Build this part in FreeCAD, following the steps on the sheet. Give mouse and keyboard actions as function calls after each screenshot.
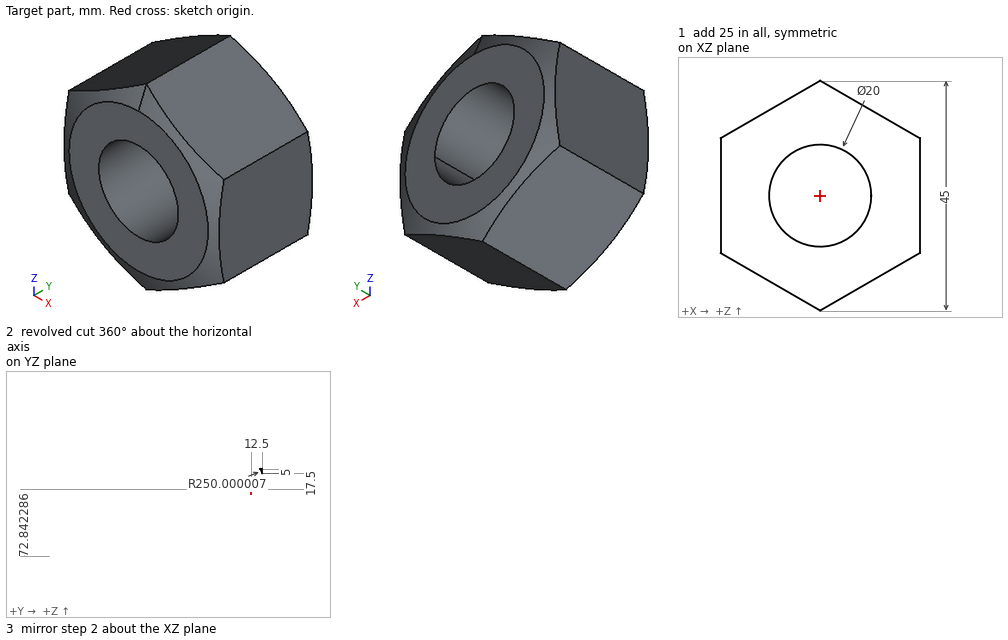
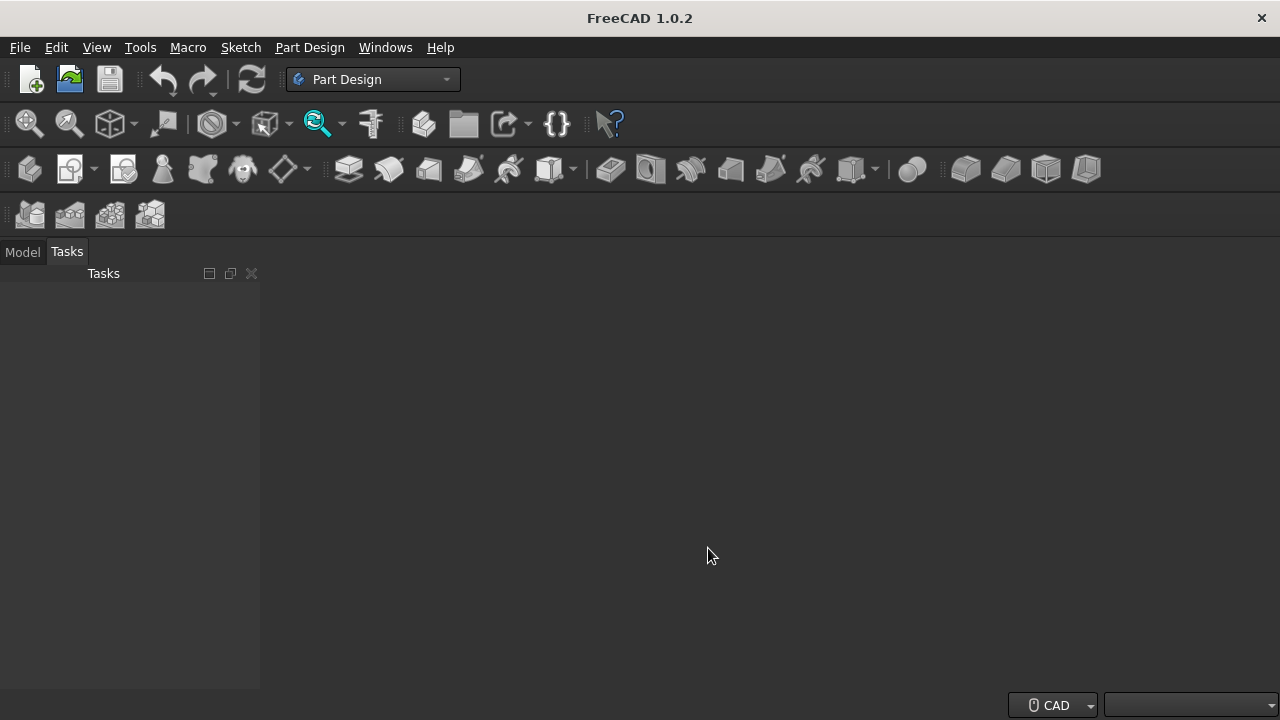
click(30, 80)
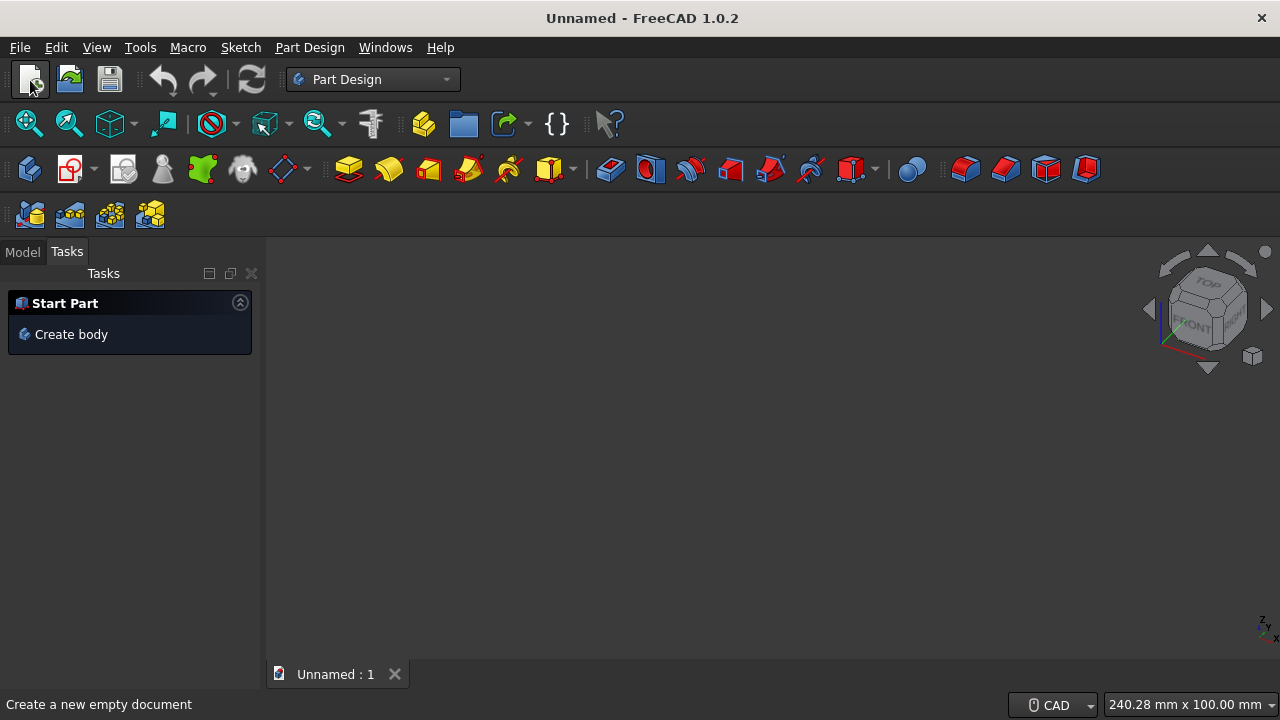
click(70, 170)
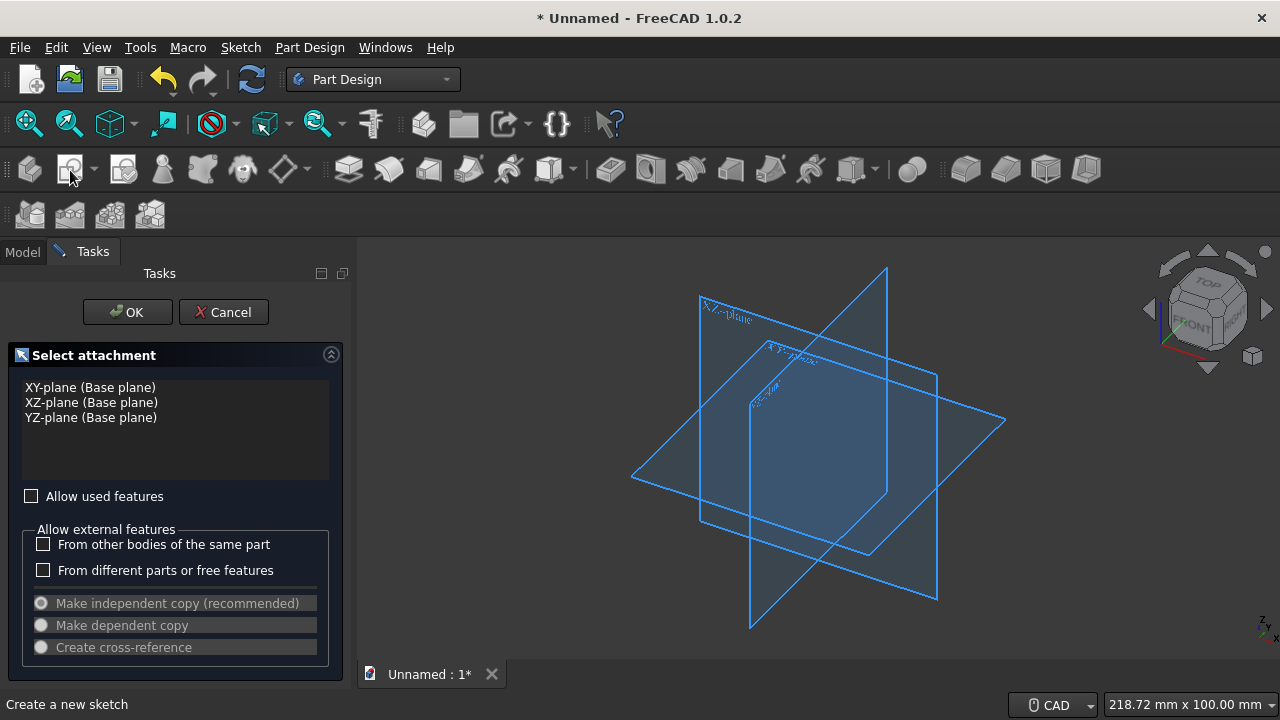
click(82, 402)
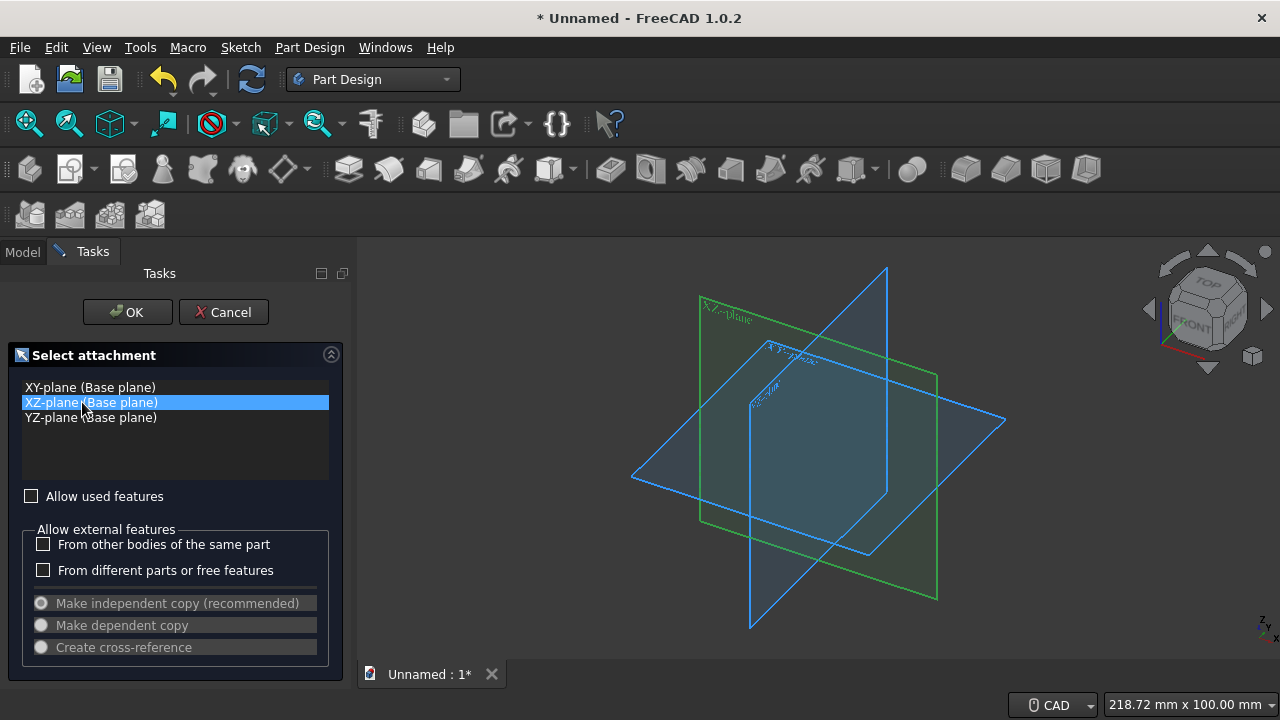
click(128, 312)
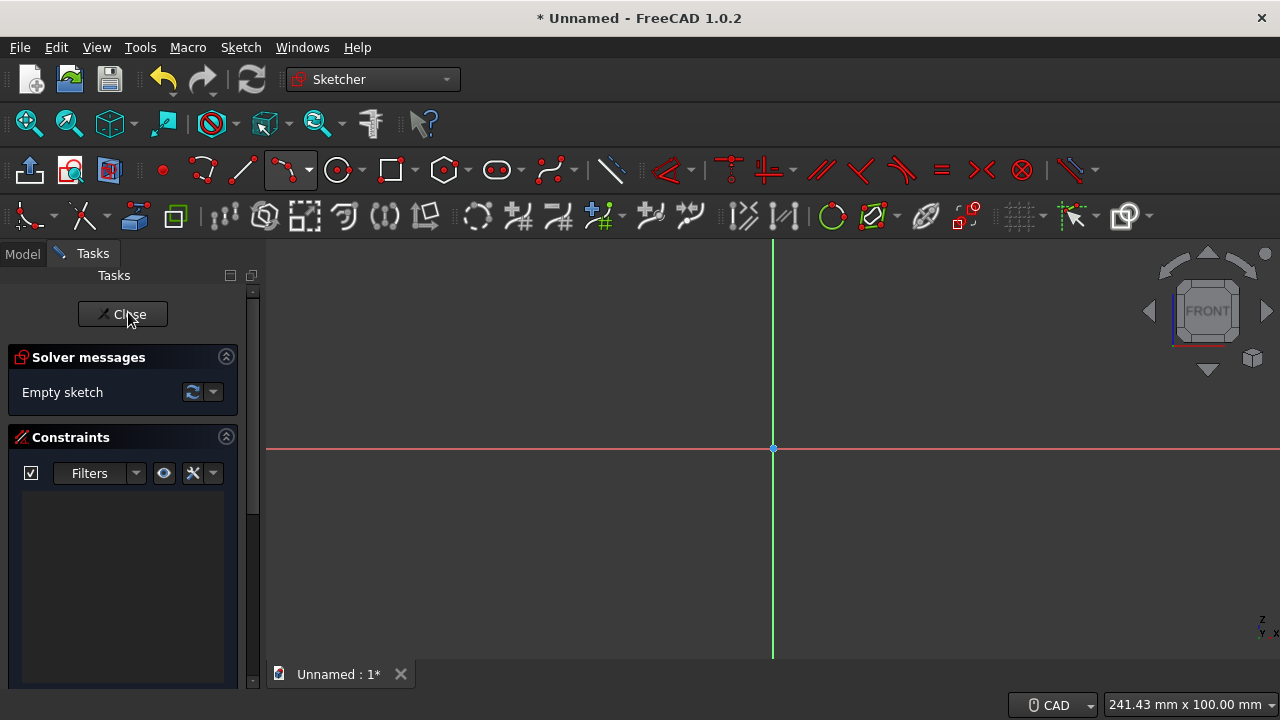
scroll(912, 449, up, 2)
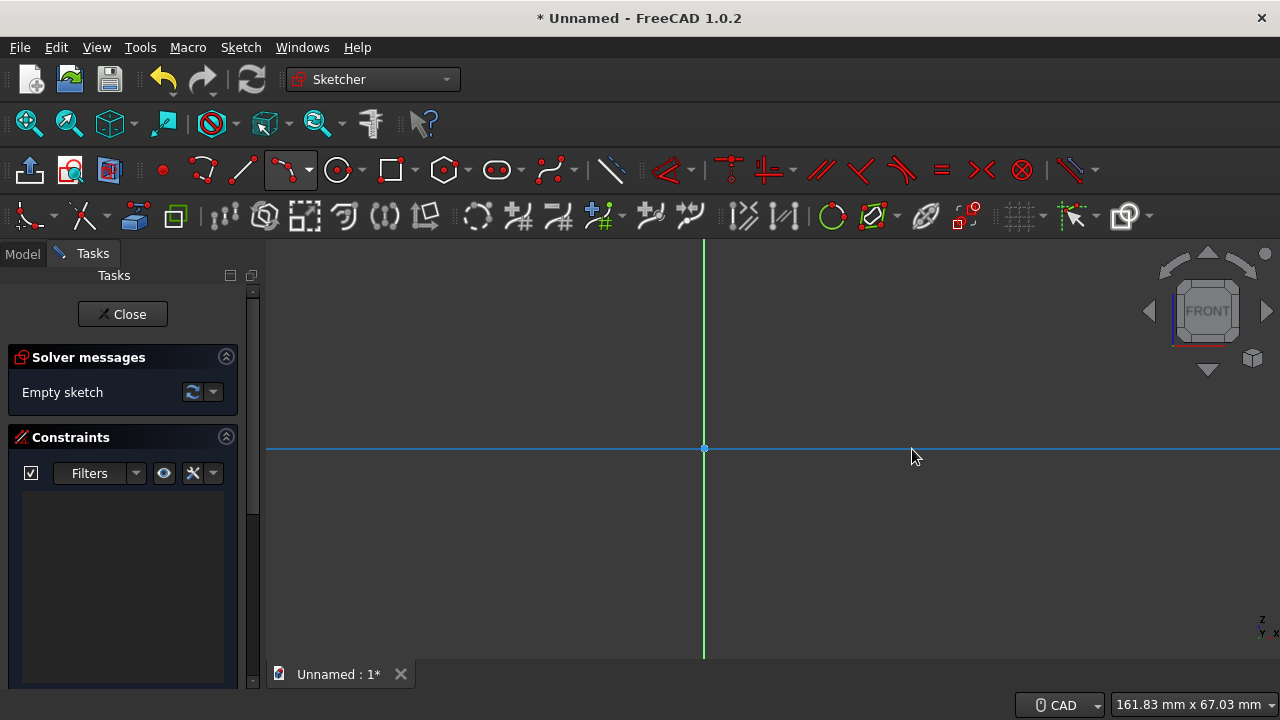
click(444, 170)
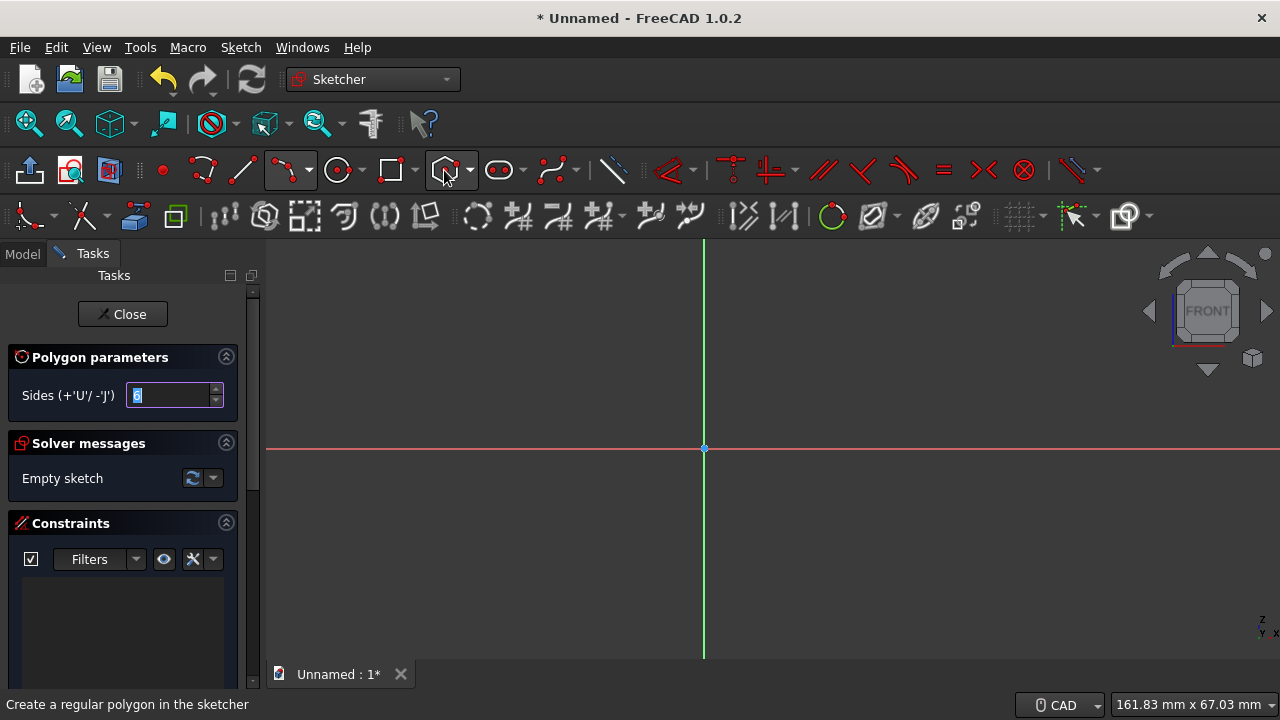
click(704, 449)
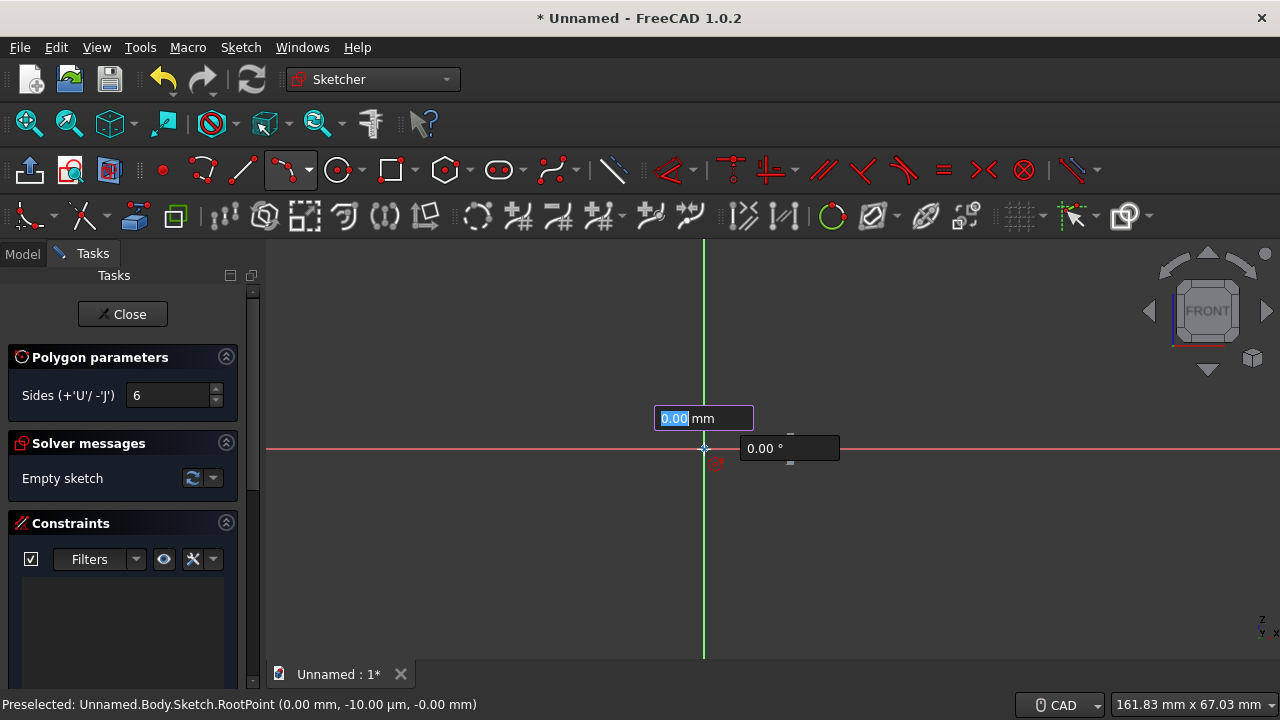
click(704, 590)
right_click(704, 590)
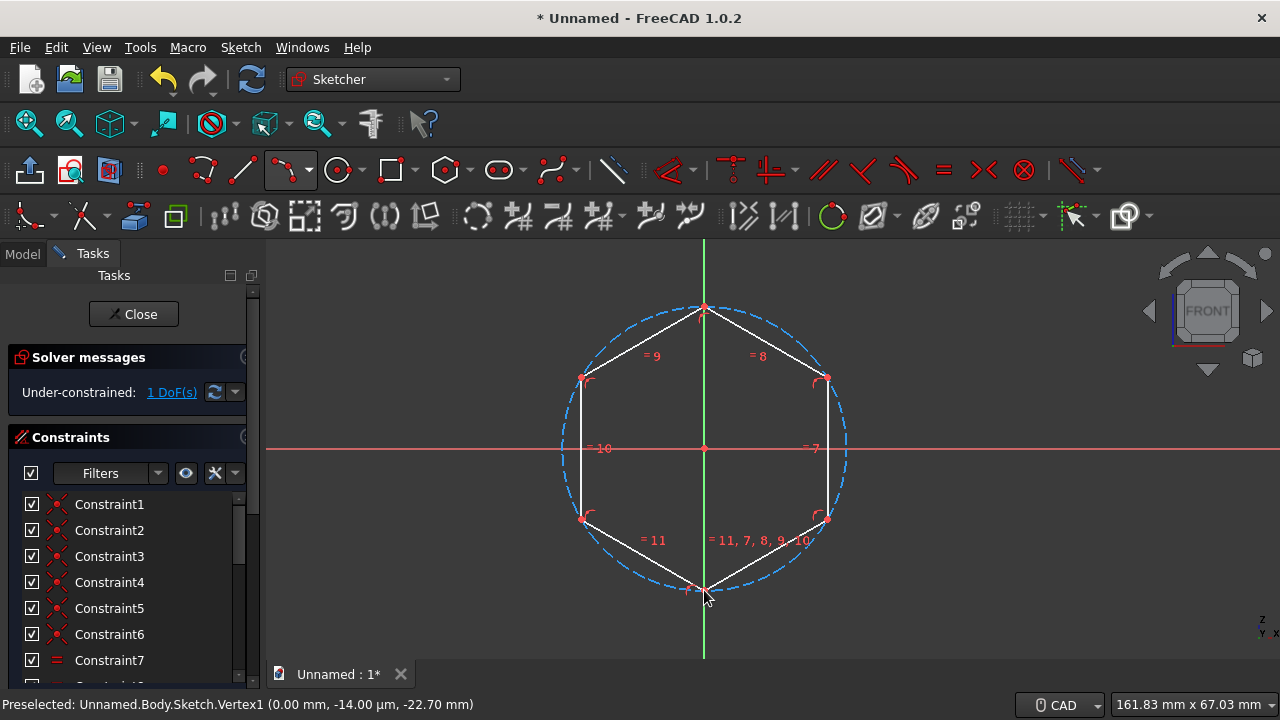
click(338, 170)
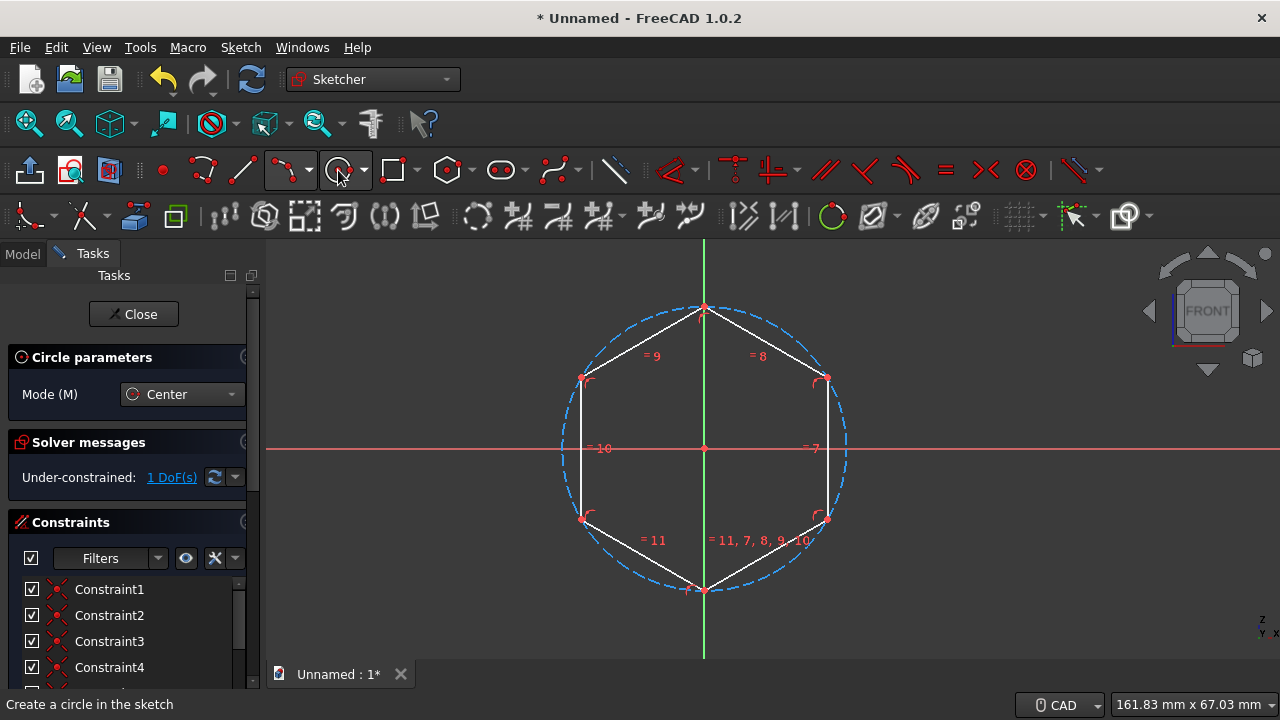
click(704, 449)
click(749, 404)
key(Escape)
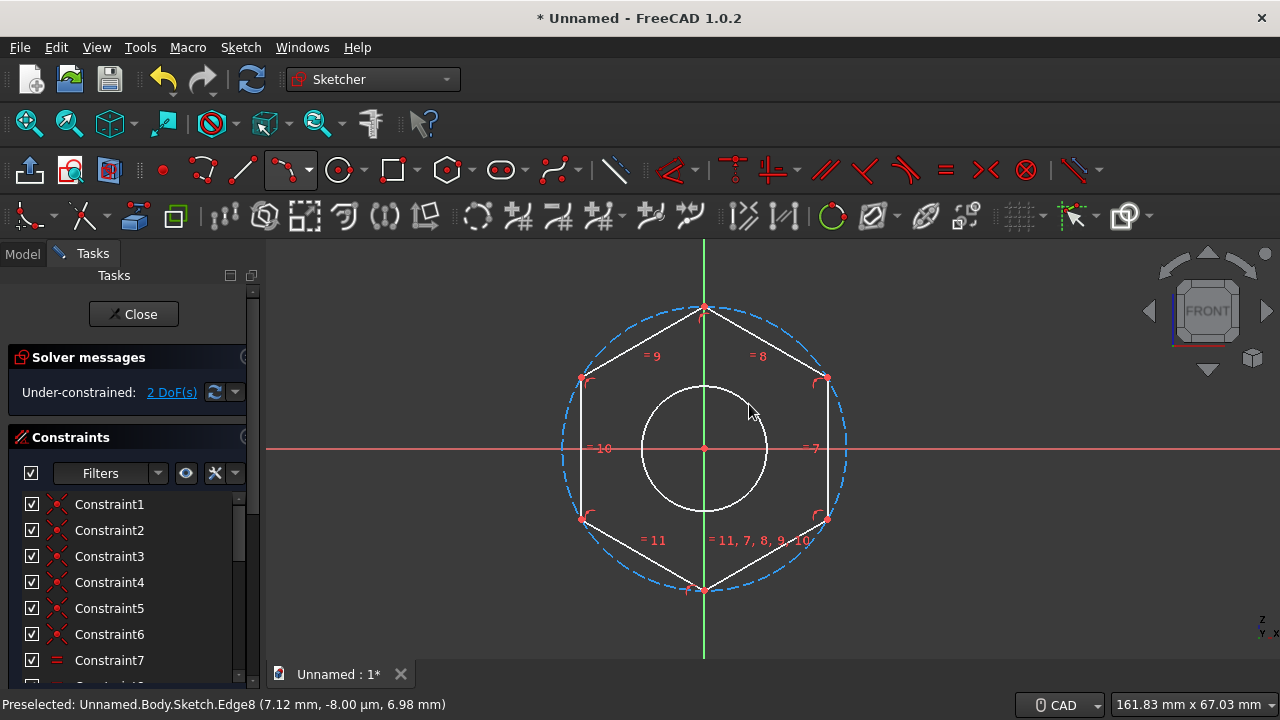
click(748, 404)